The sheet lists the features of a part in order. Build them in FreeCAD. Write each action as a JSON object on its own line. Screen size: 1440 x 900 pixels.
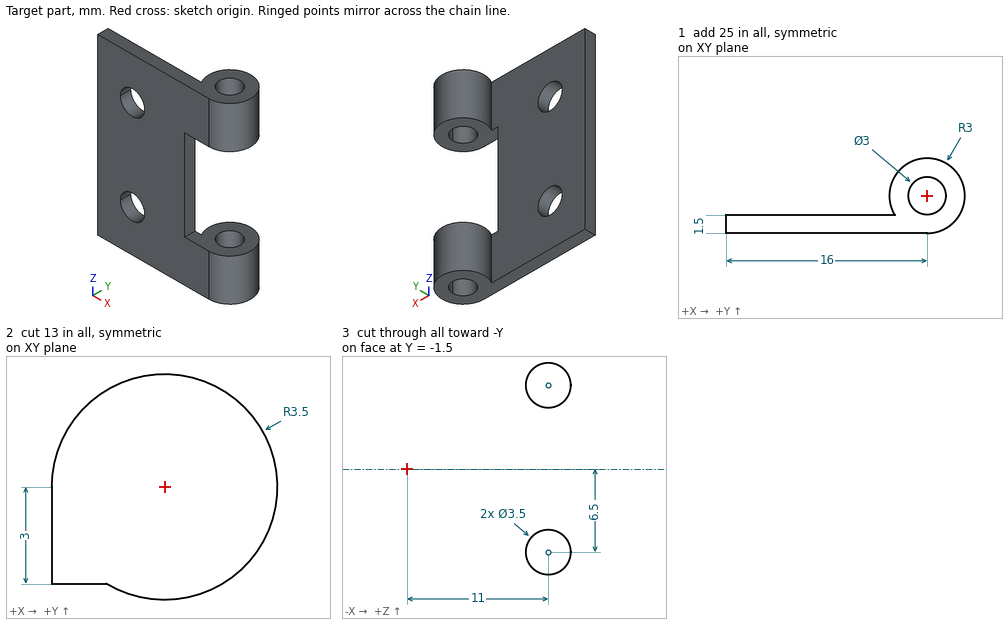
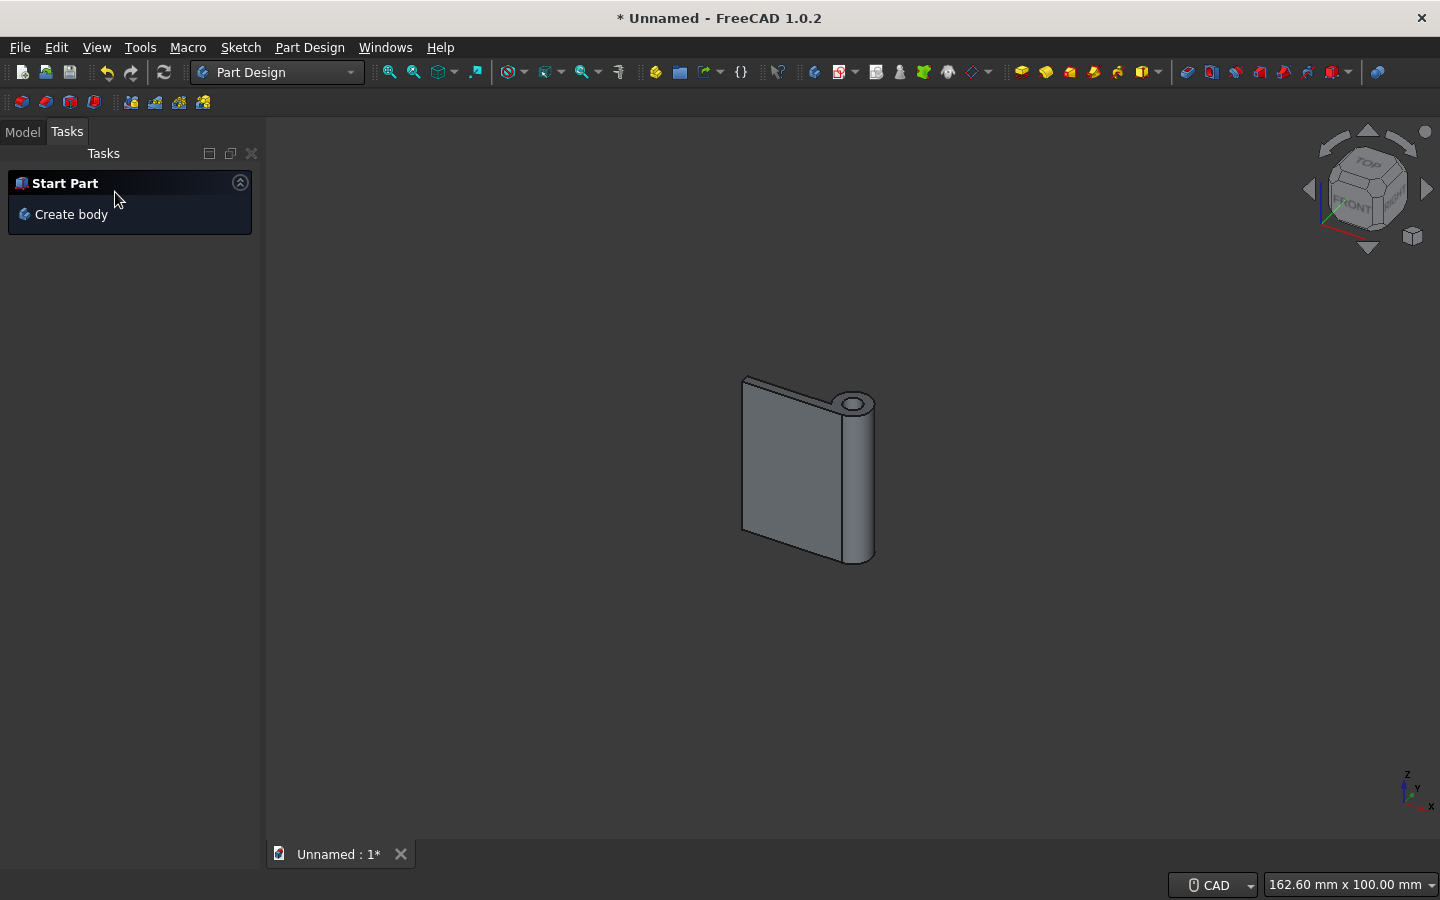
{"action": "left_click", "coordinate": [390, 72]}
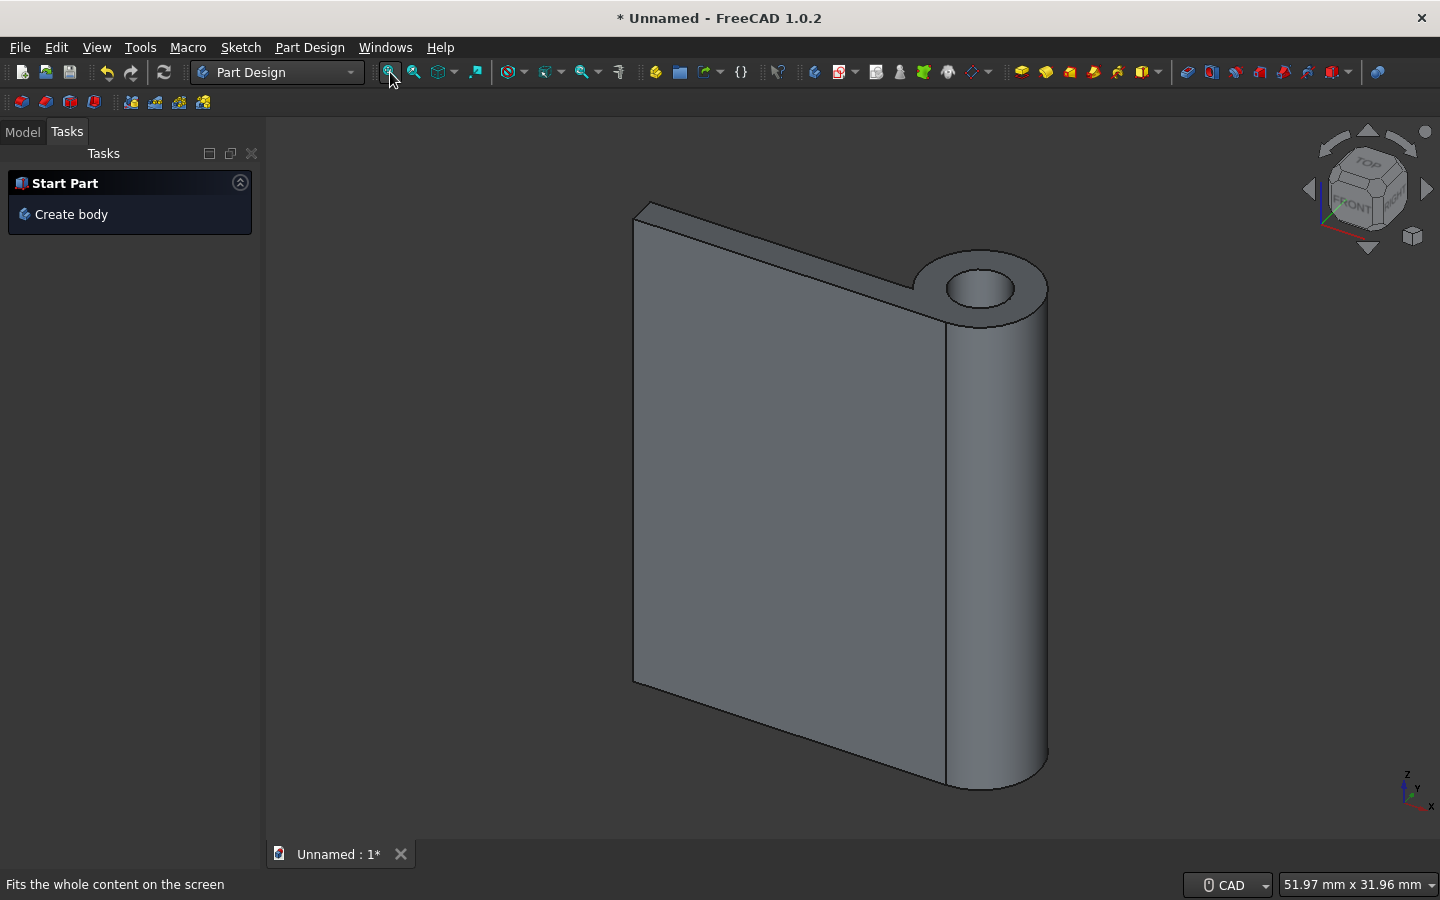
{"action": "left_click", "coordinate": [840, 72]}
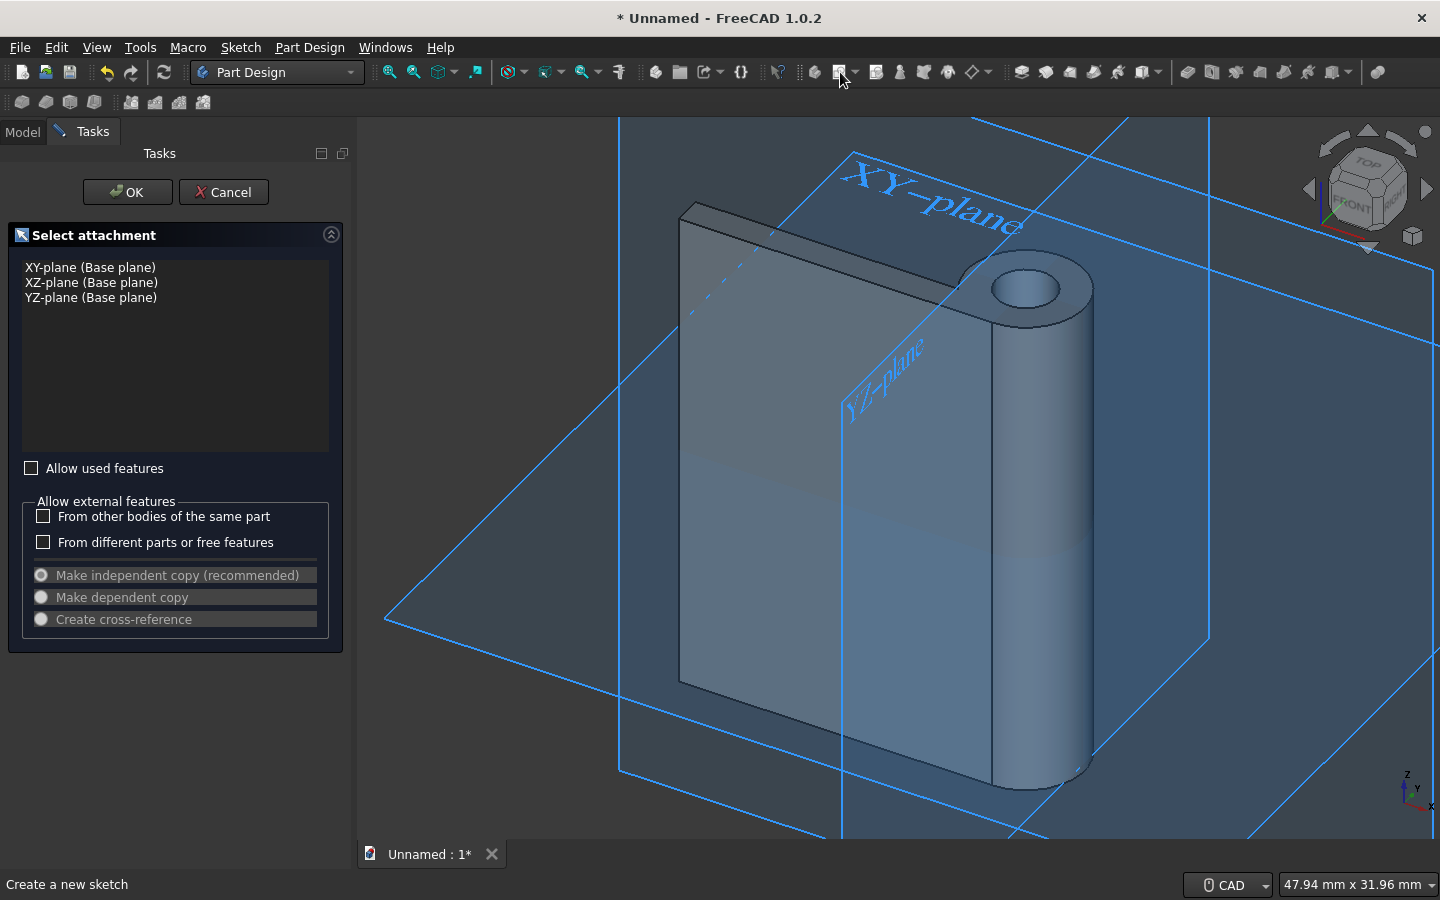
{"action": "left_click", "coordinate": [82, 268]}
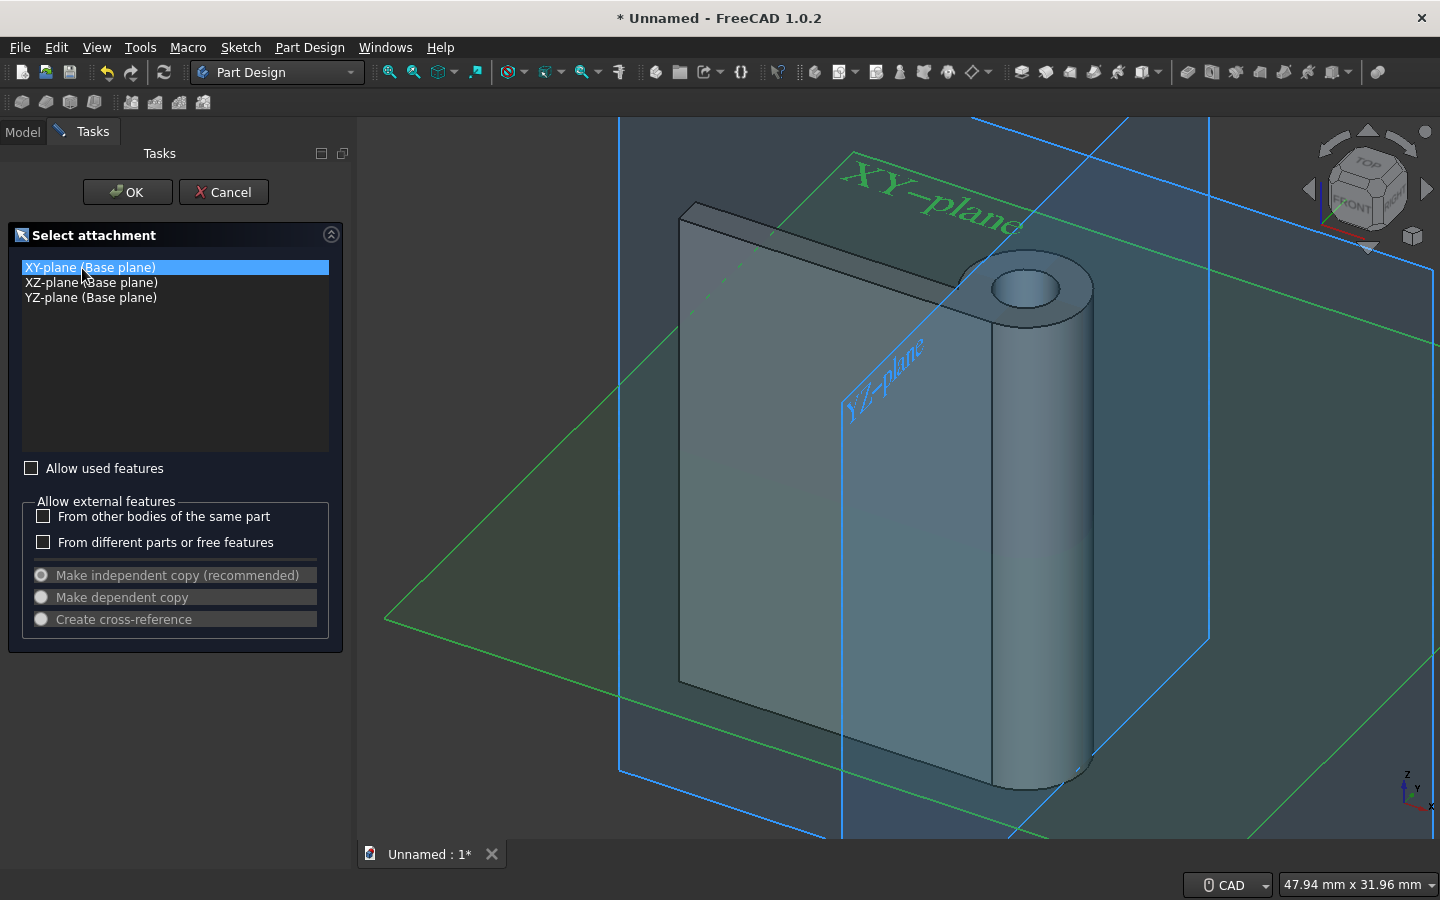
{"action": "left_click", "coordinate": [128, 192]}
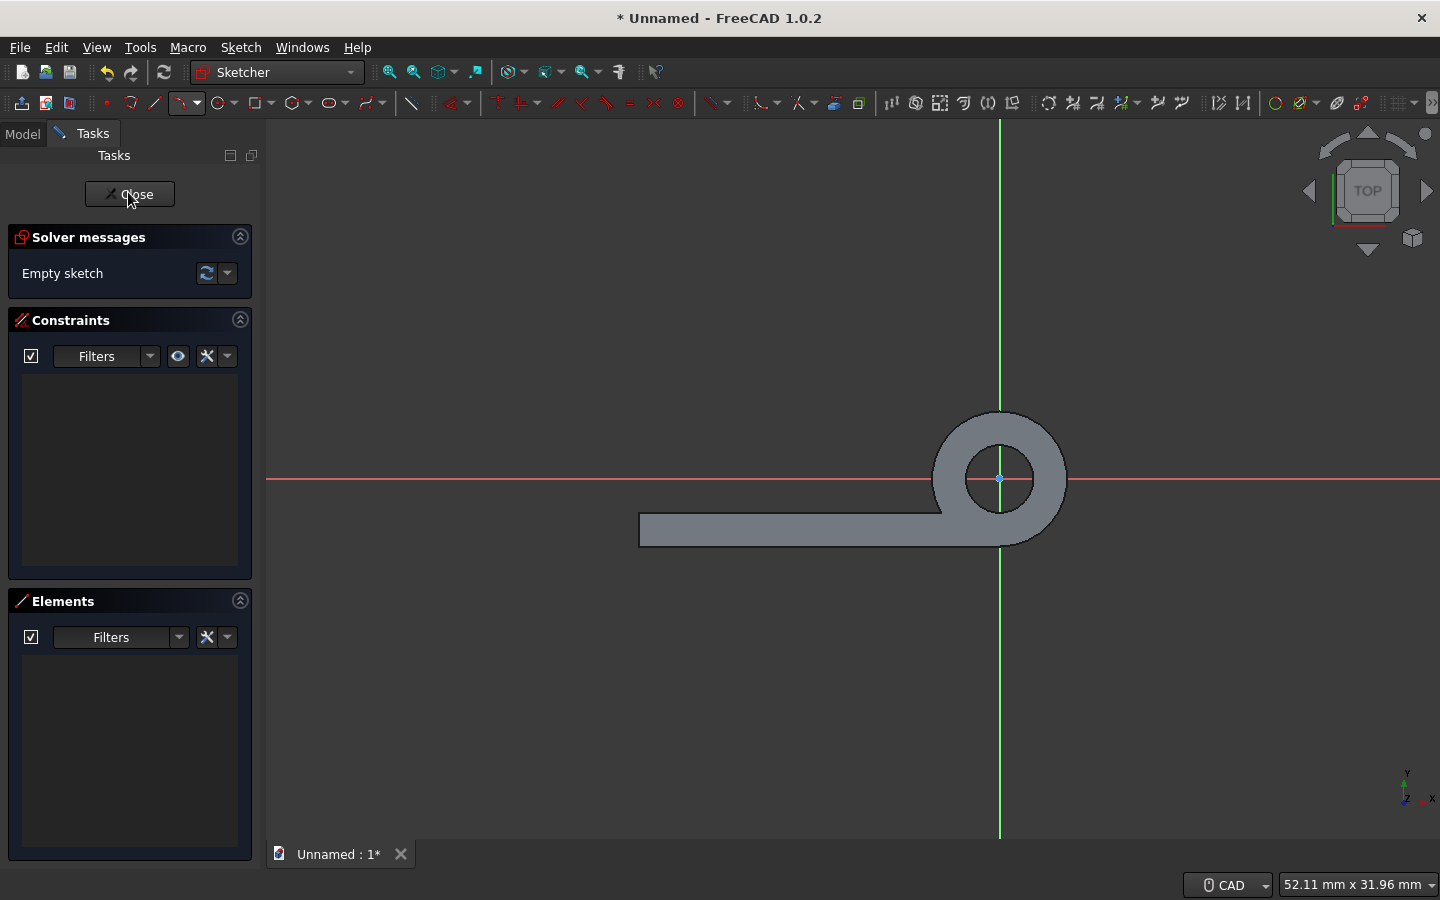
{"action": "left_click", "coordinate": [70, 104]}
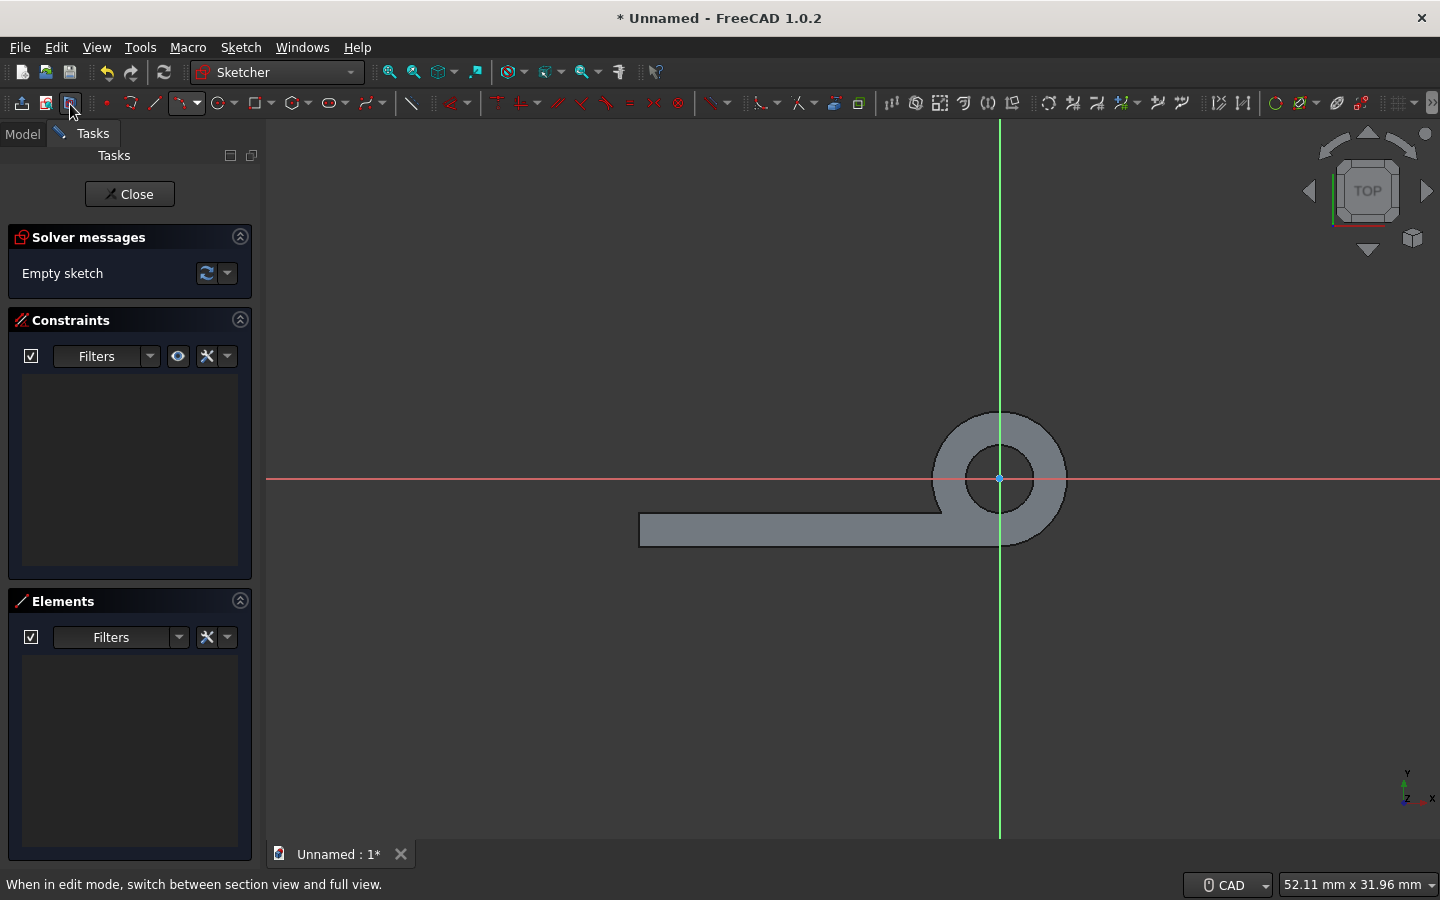
{"action": "scroll", "coordinate": [1063, 498], "scroll_direction": "up", "scroll_amount": 7}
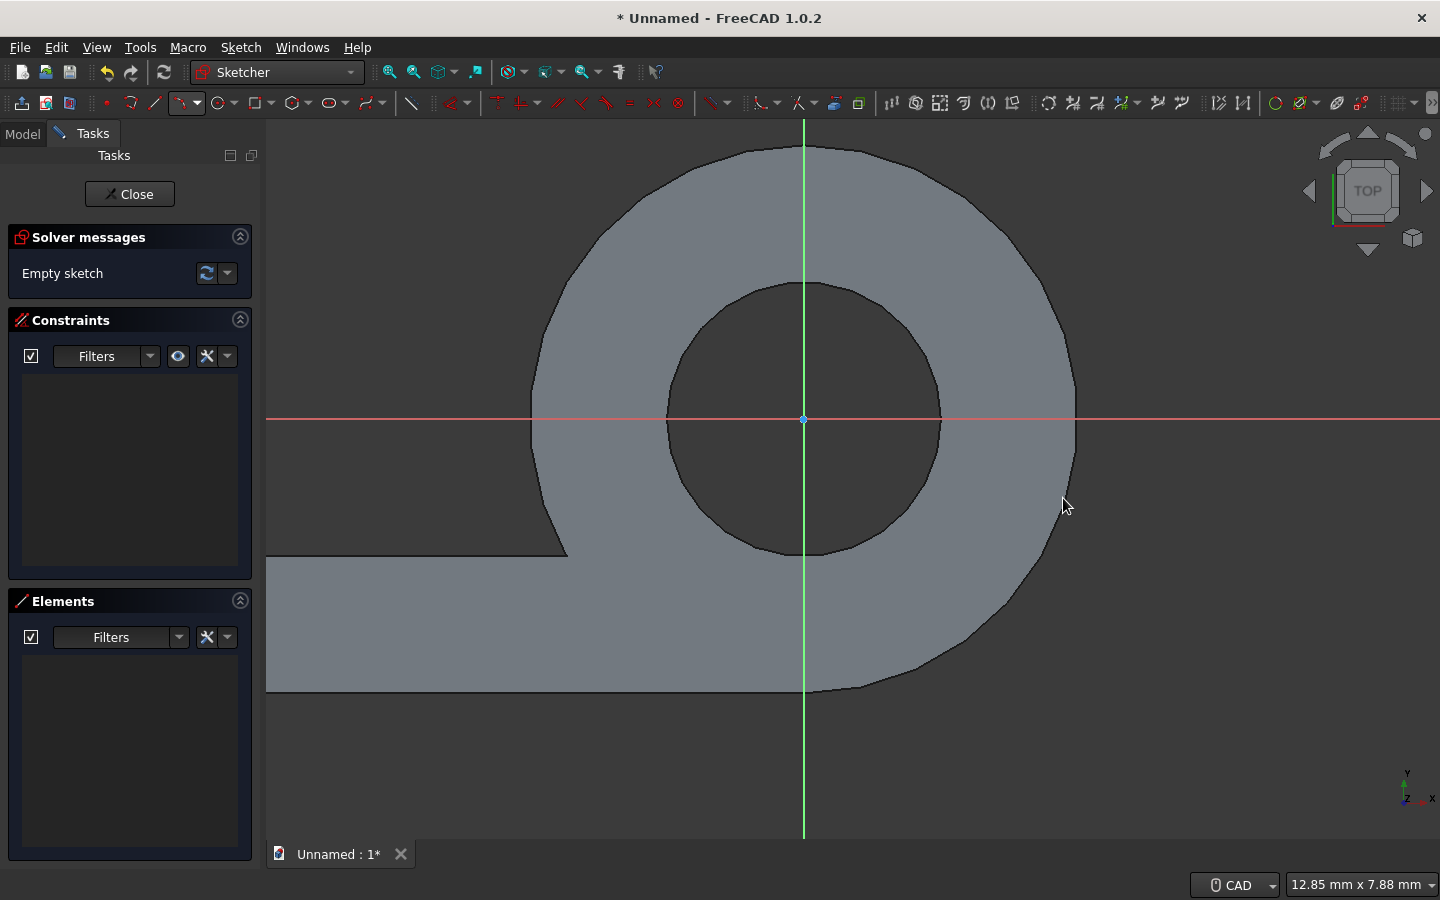
{"action": "left_click", "coordinate": [132, 104]}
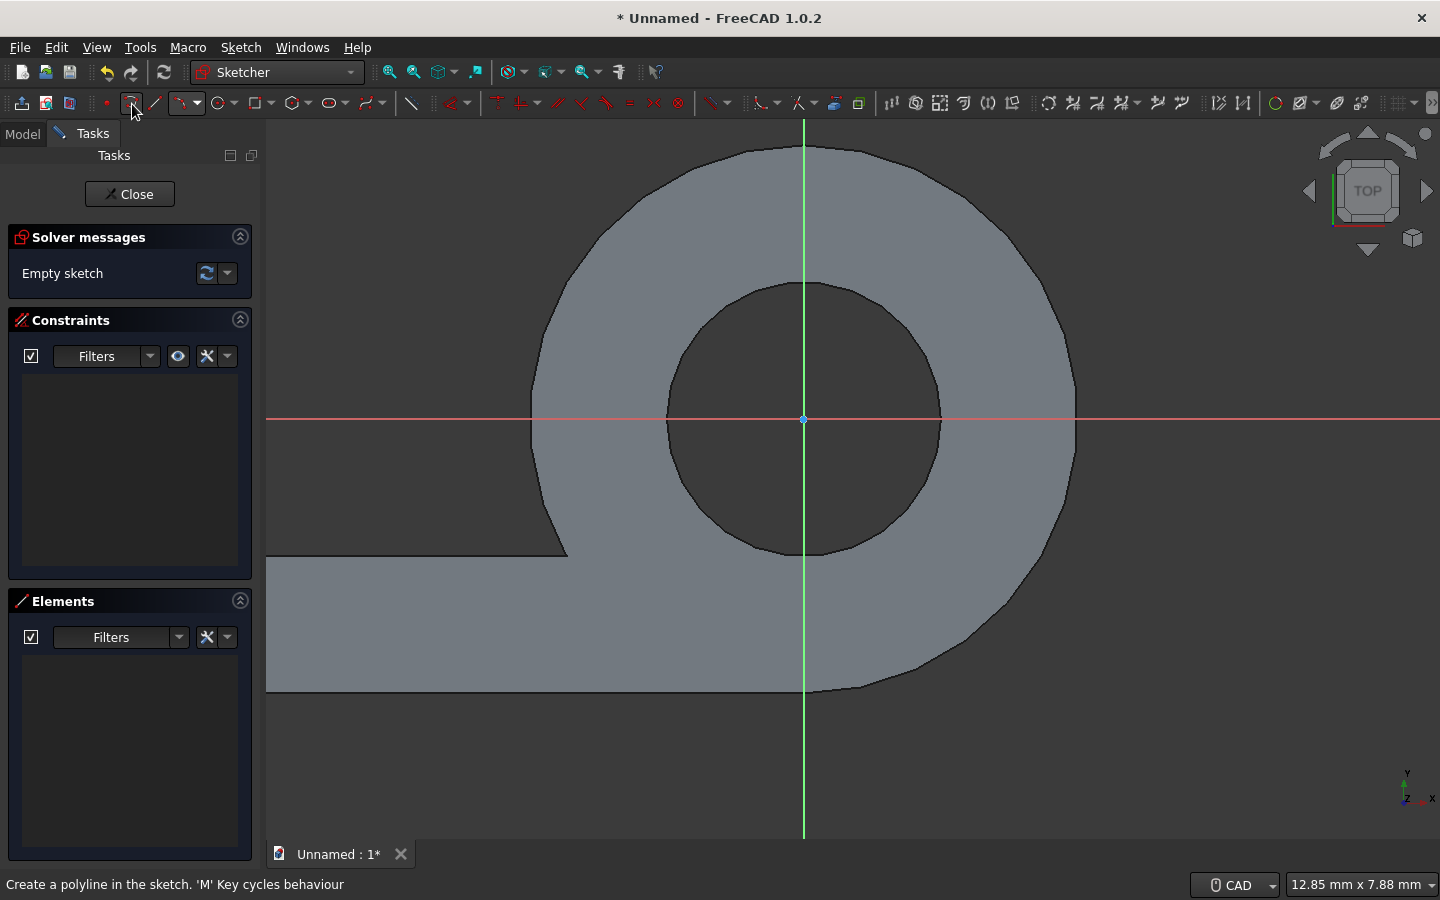
{"action": "left_click", "coordinate": [484, 419]}
{"action": "left_click", "coordinate": [484, 693]}
{"action": "left_click", "coordinate": [639, 693]}
{"action": "right_click", "coordinate": [639, 693]}